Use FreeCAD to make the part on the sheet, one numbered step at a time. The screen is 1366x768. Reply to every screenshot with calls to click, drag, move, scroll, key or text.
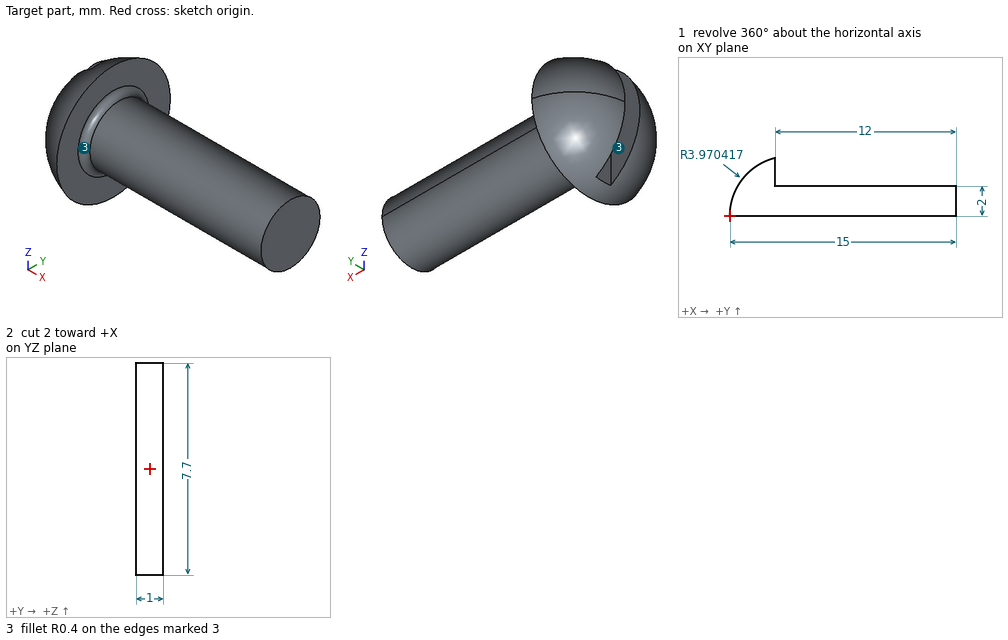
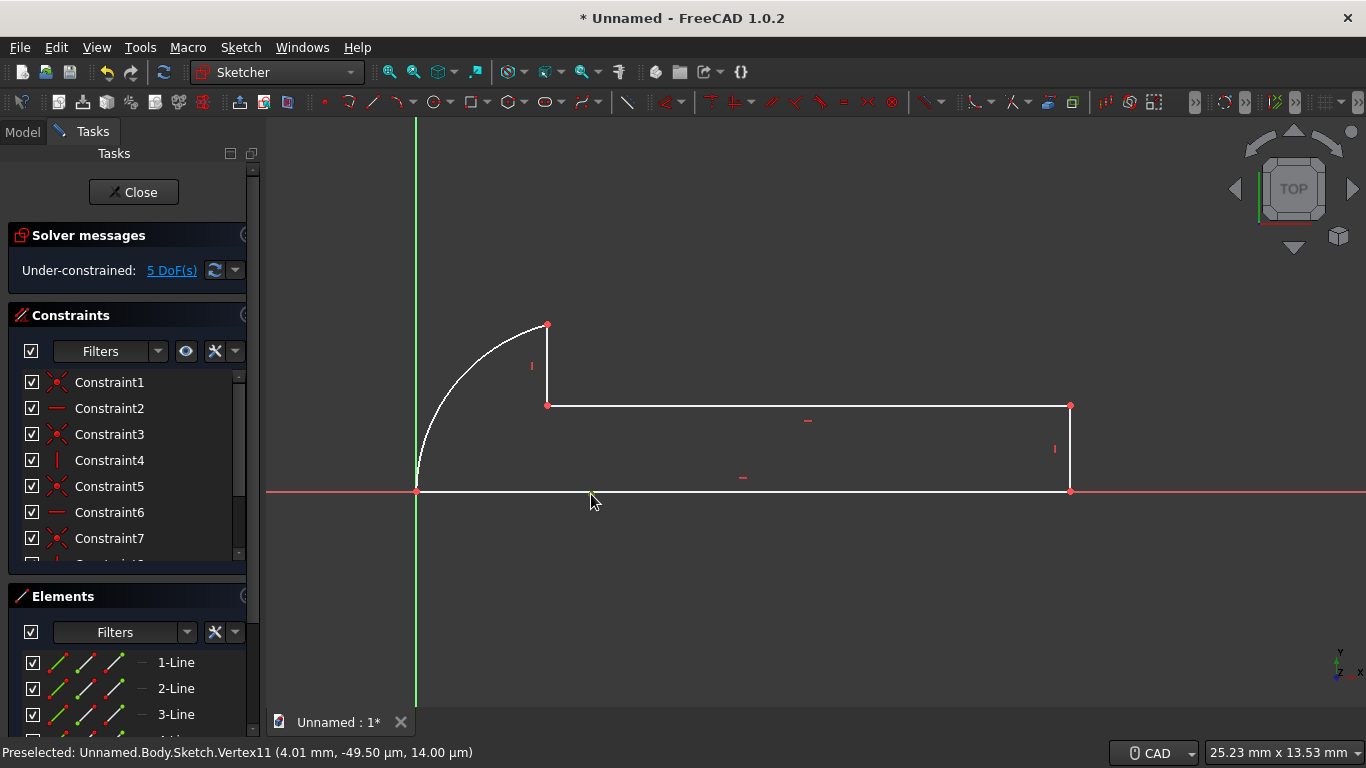
click(359, 492)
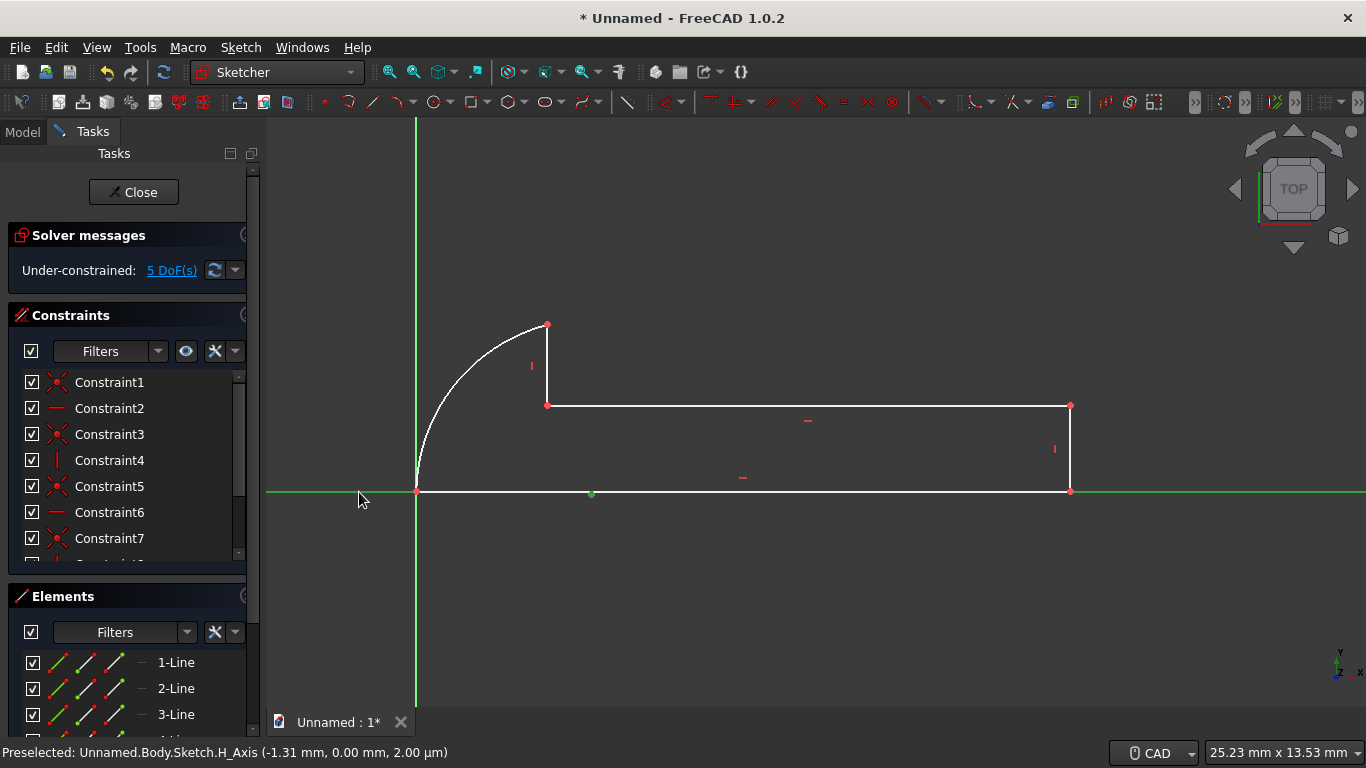
key(c)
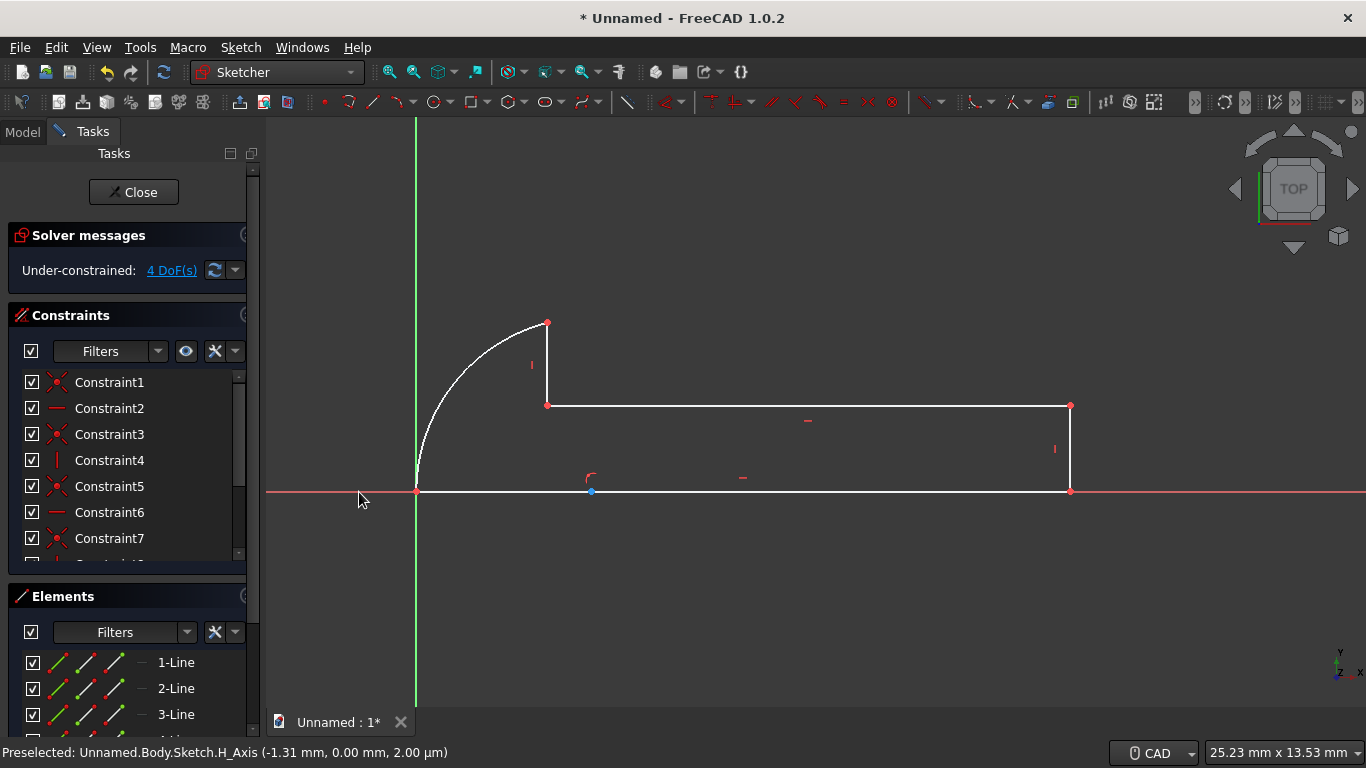
click(666, 102)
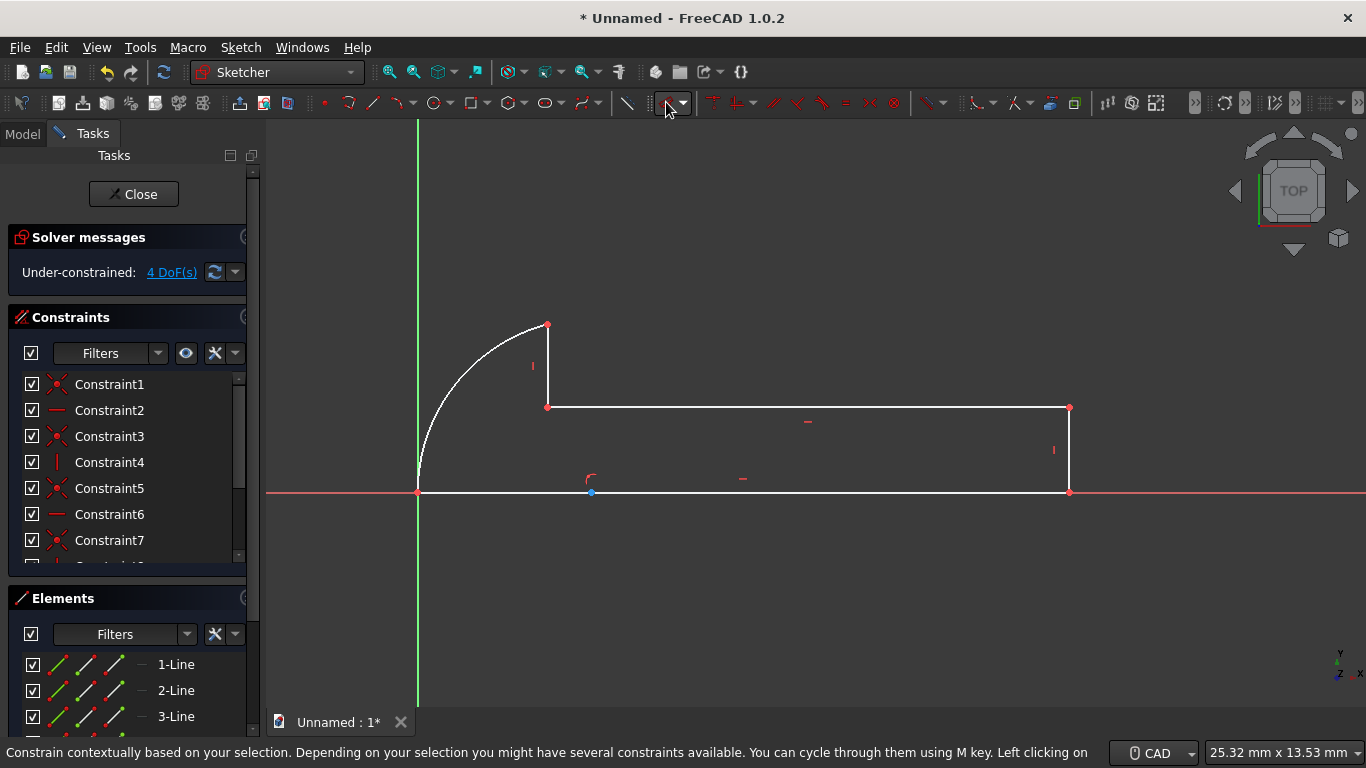
click(486, 354)
click(467, 329)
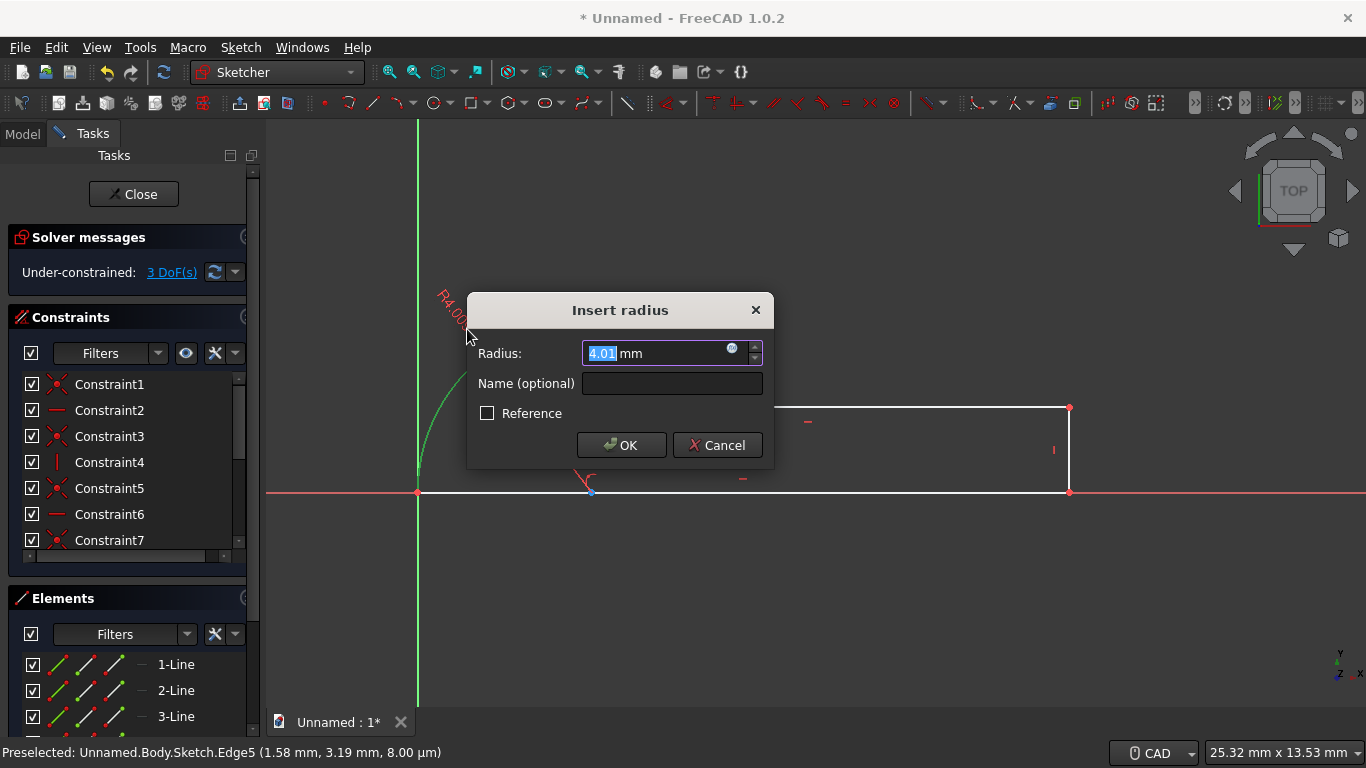
text(3.970417)
key(Return)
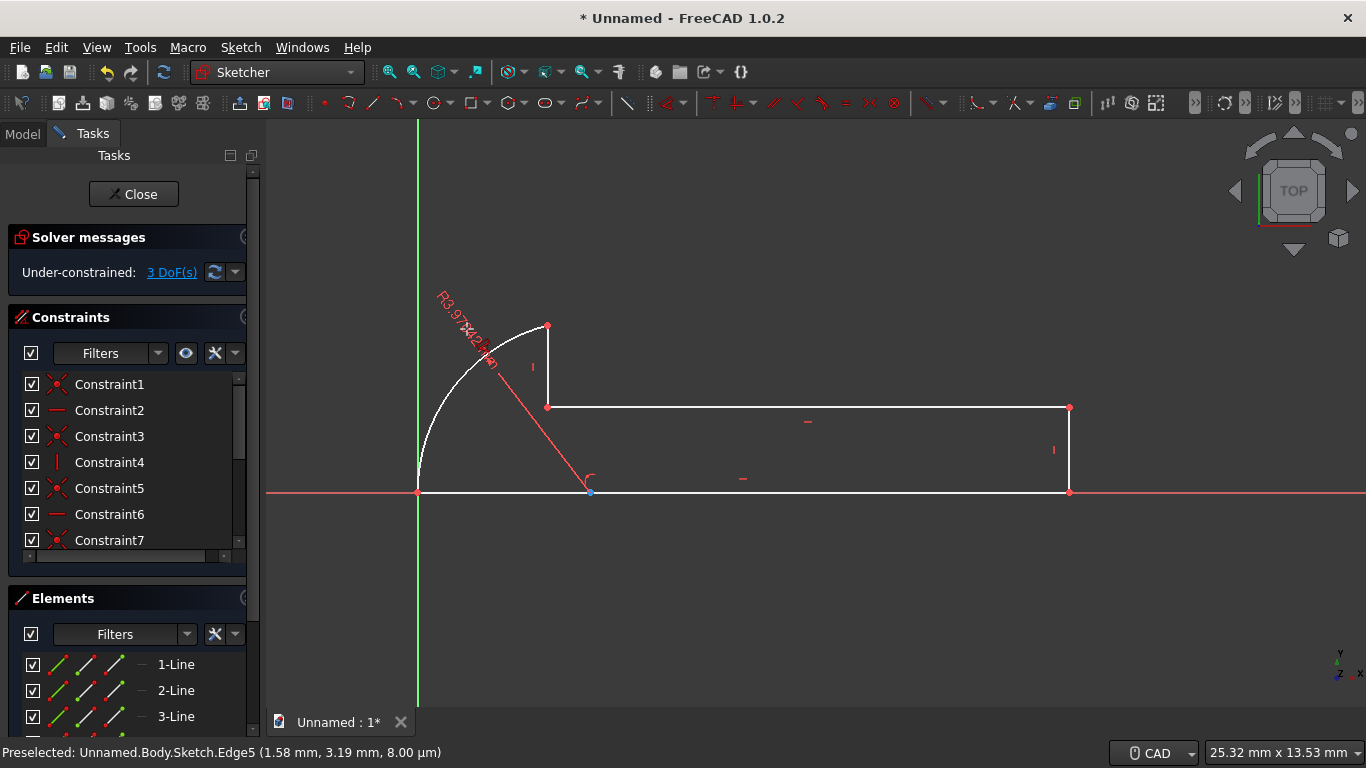
click(1069, 467)
click(1103, 450)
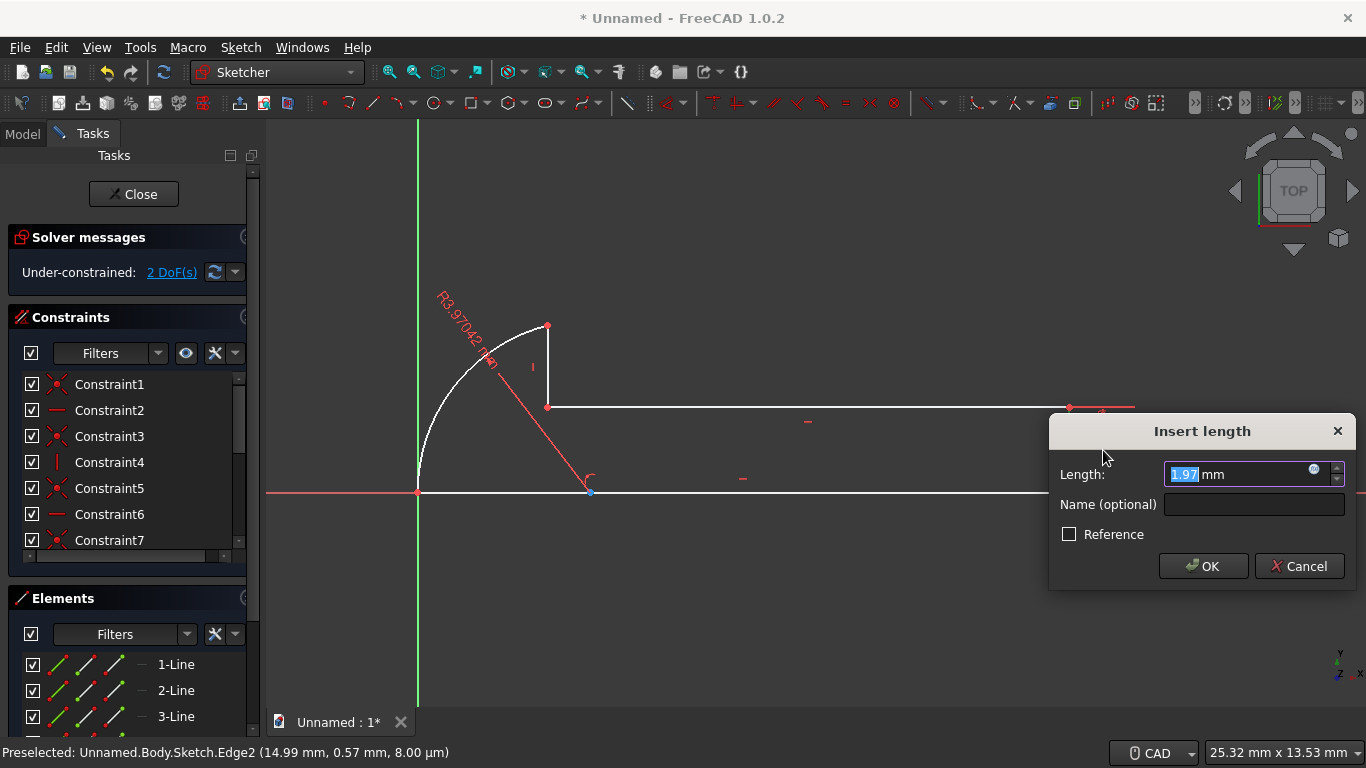
text(2)
key(Return)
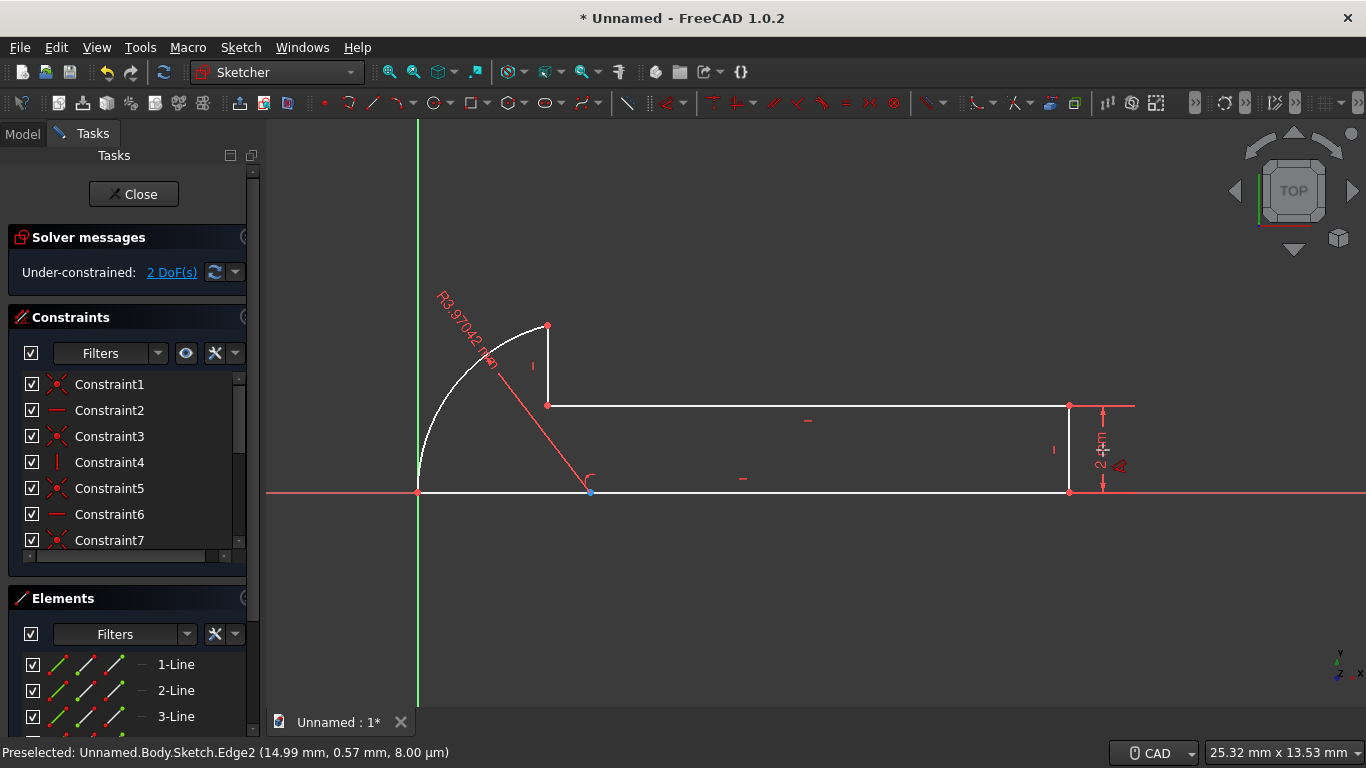
click(613, 493)
click(743, 527)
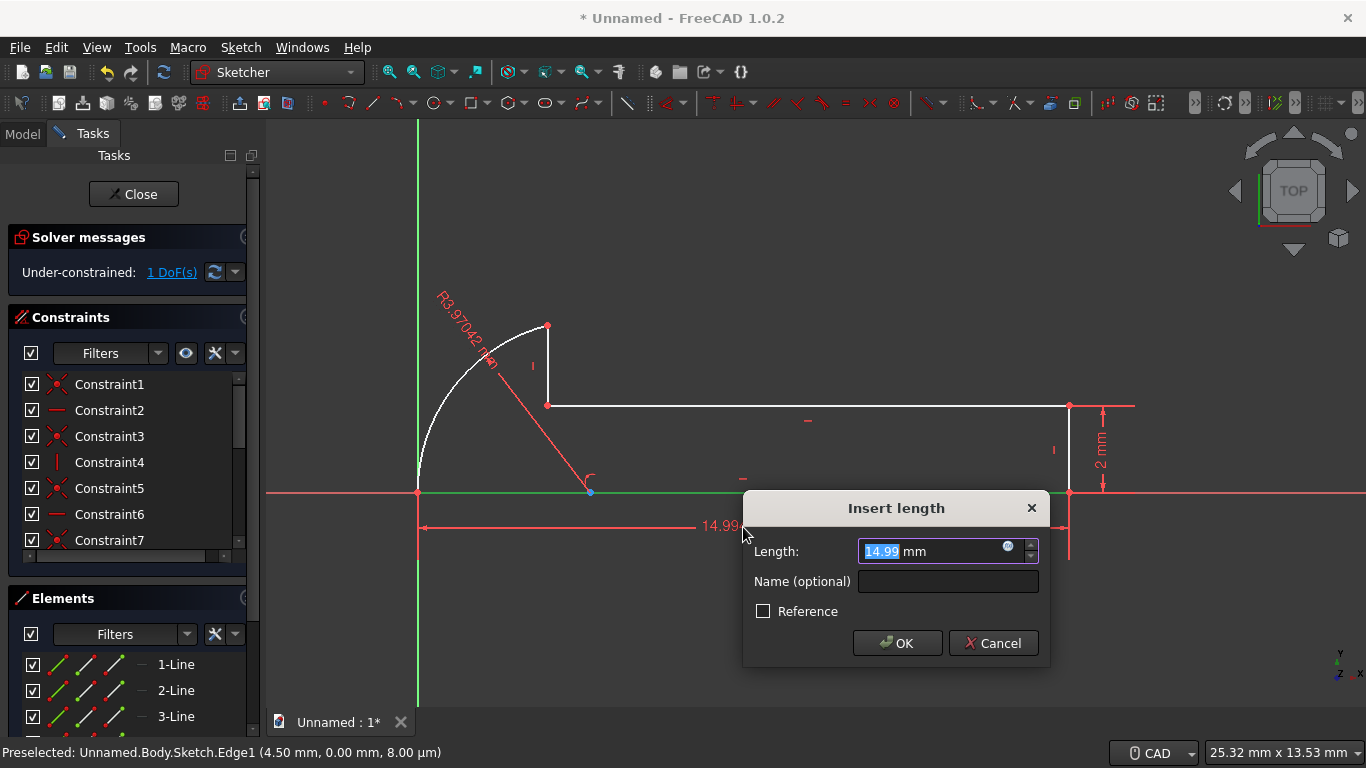
text(15)
key(Return)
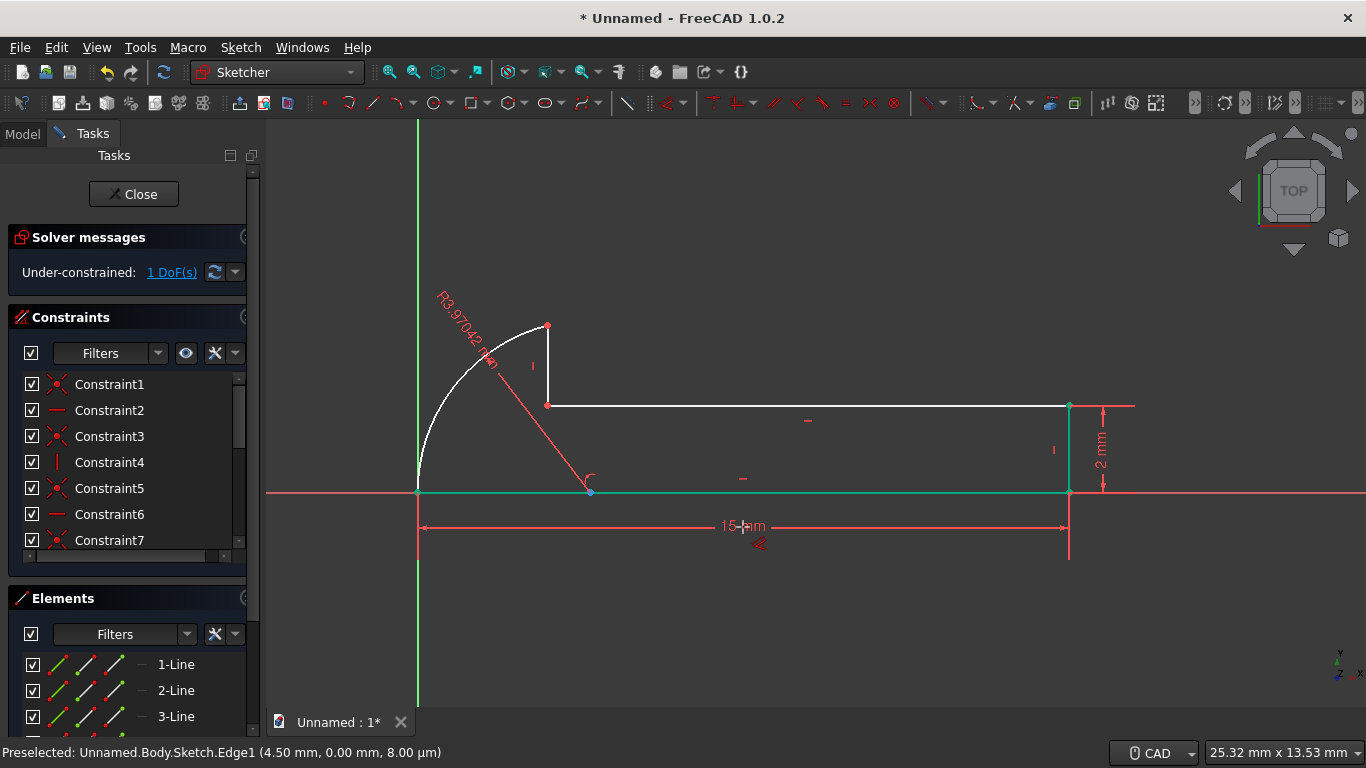
click(913, 406)
click(809, 372)